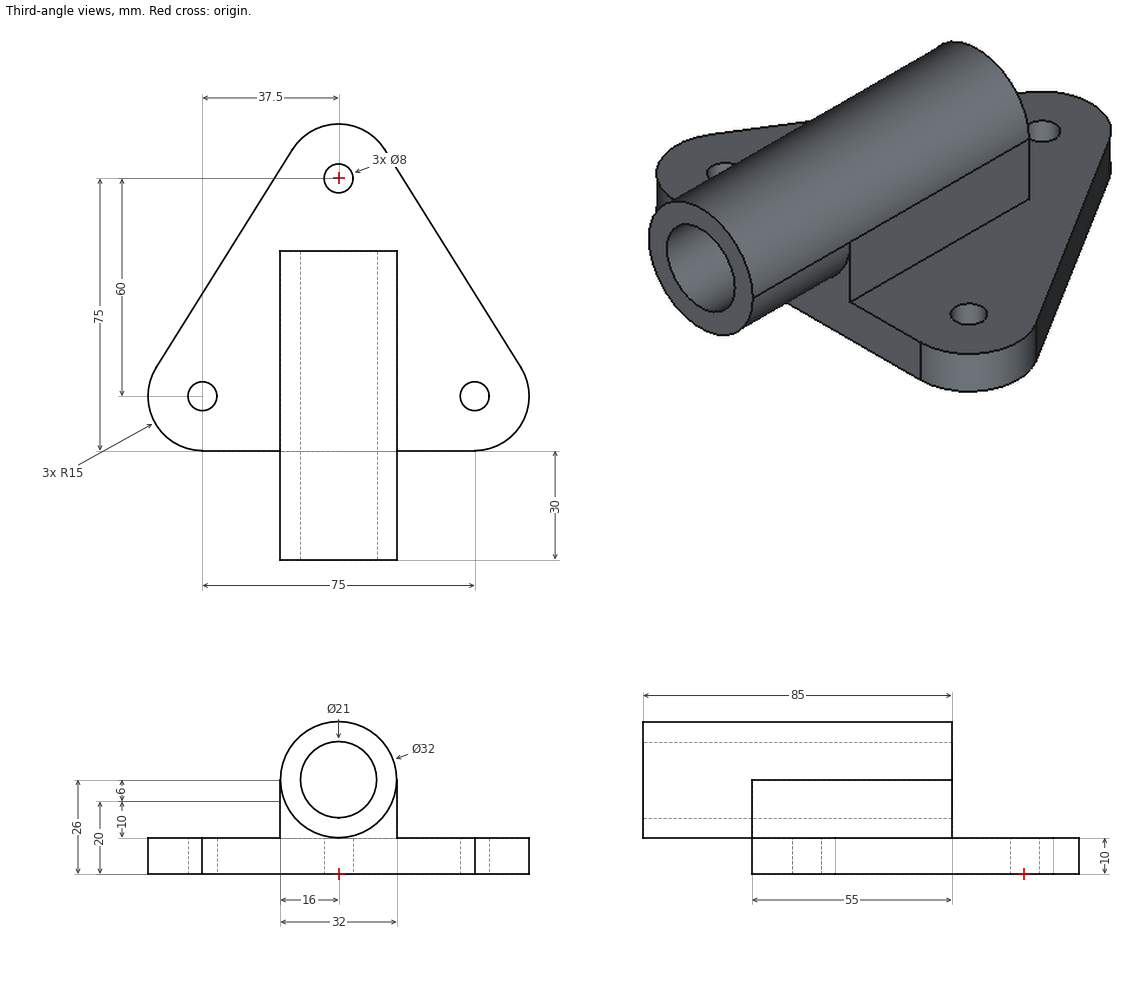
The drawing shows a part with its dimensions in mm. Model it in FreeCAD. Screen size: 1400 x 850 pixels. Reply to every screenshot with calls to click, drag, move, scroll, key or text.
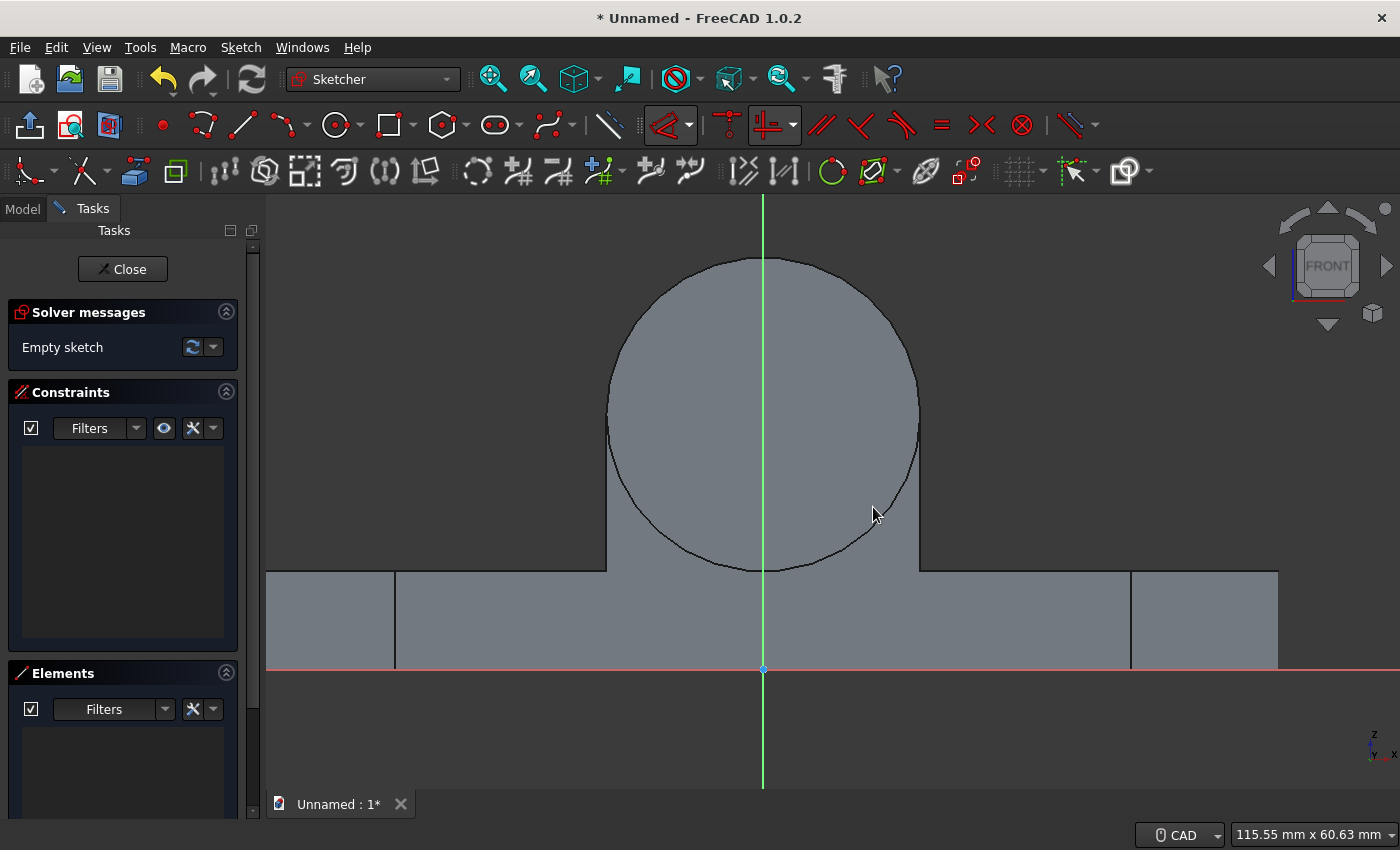
click(336, 126)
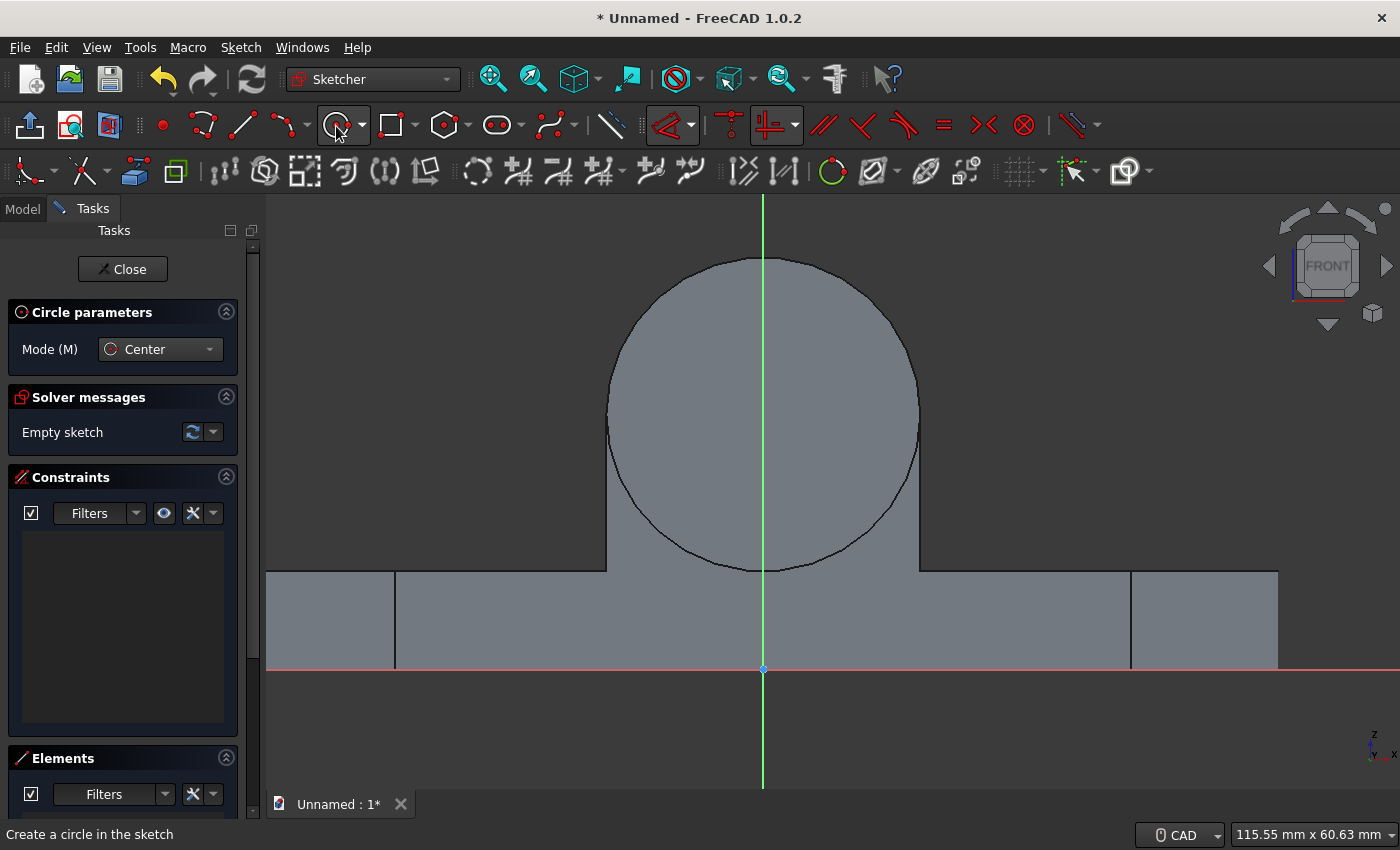
click(763, 414)
click(836, 342)
key(Escape)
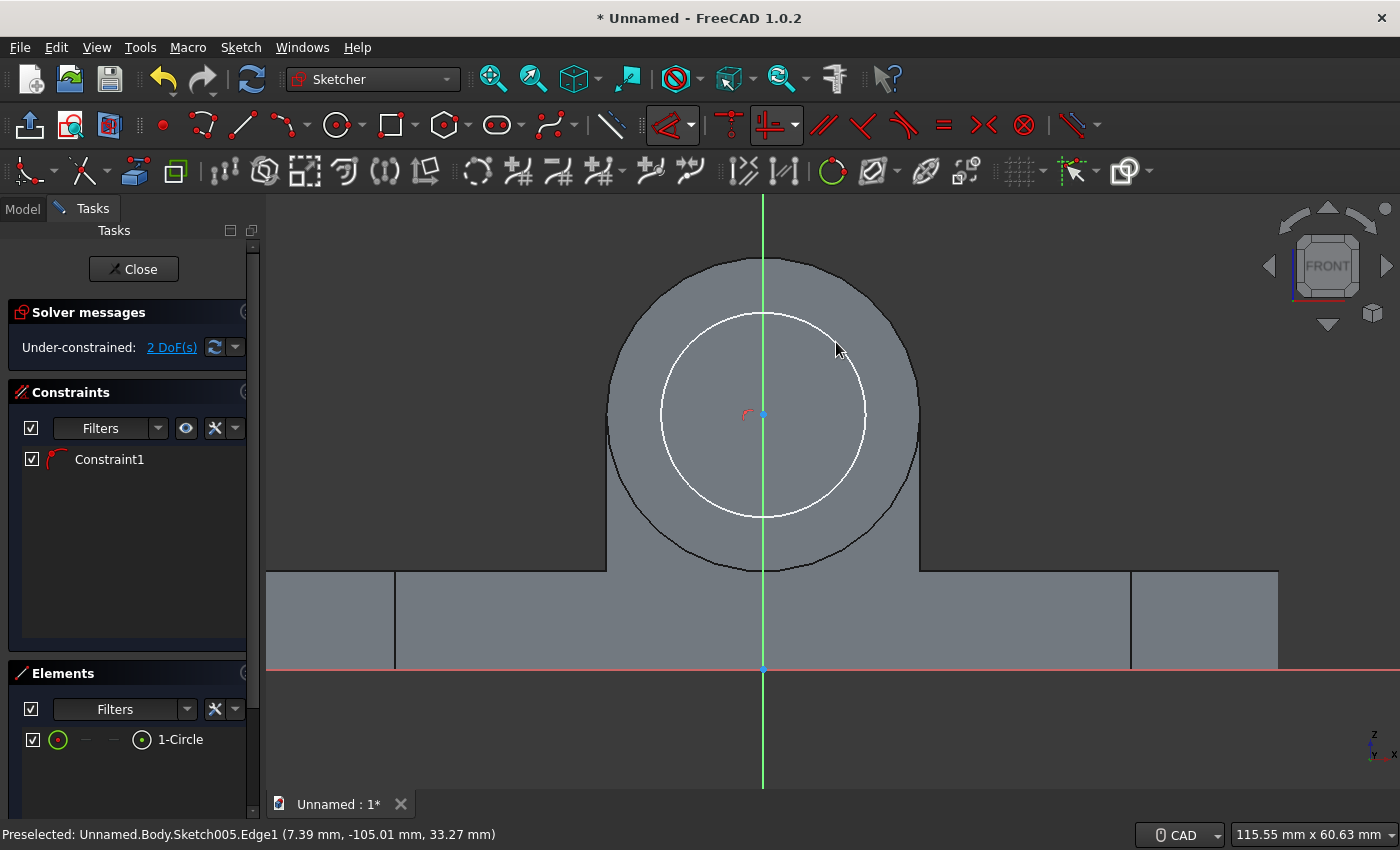
click(835, 342)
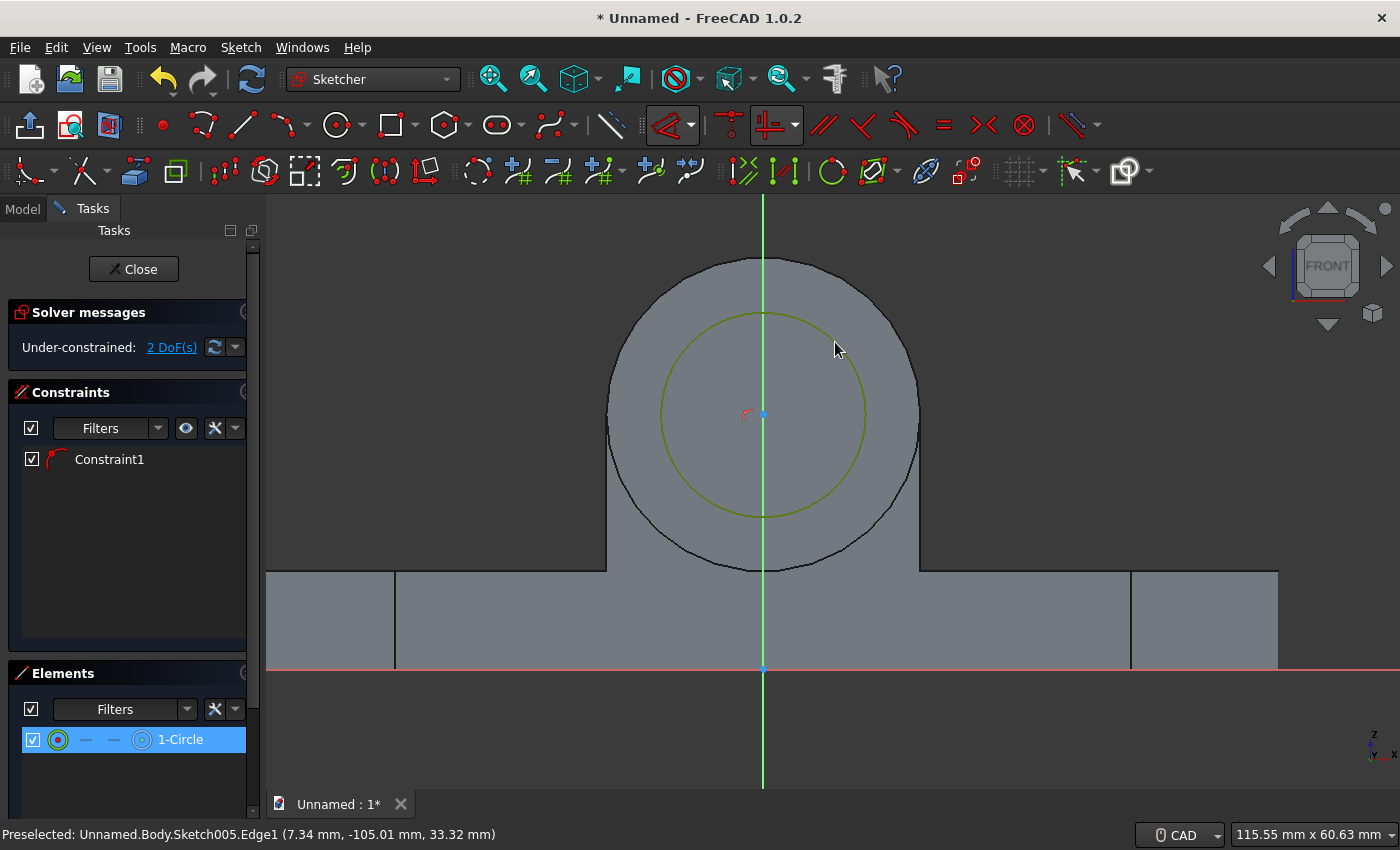
key(k)
key(o)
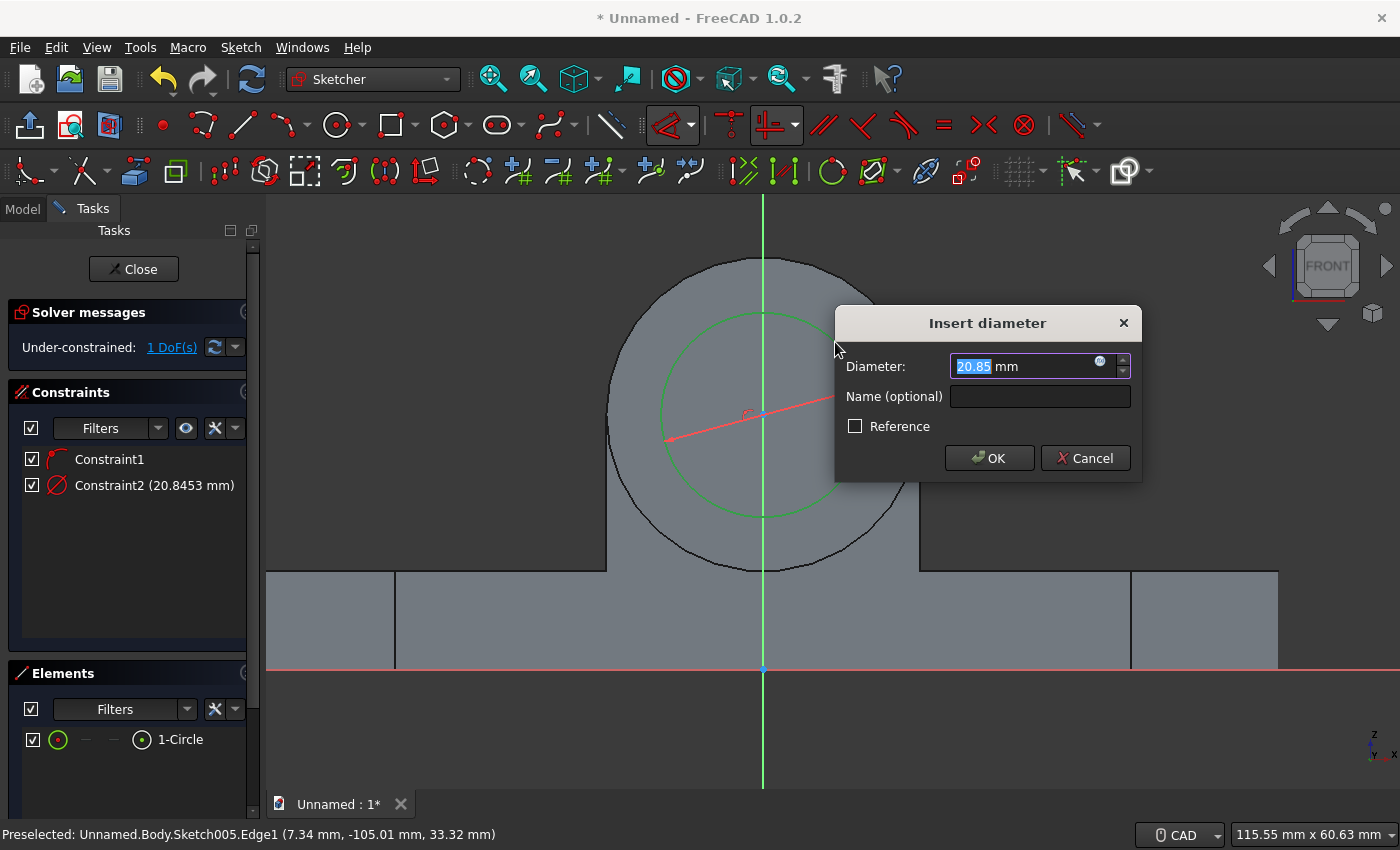
text(21)
key(Return)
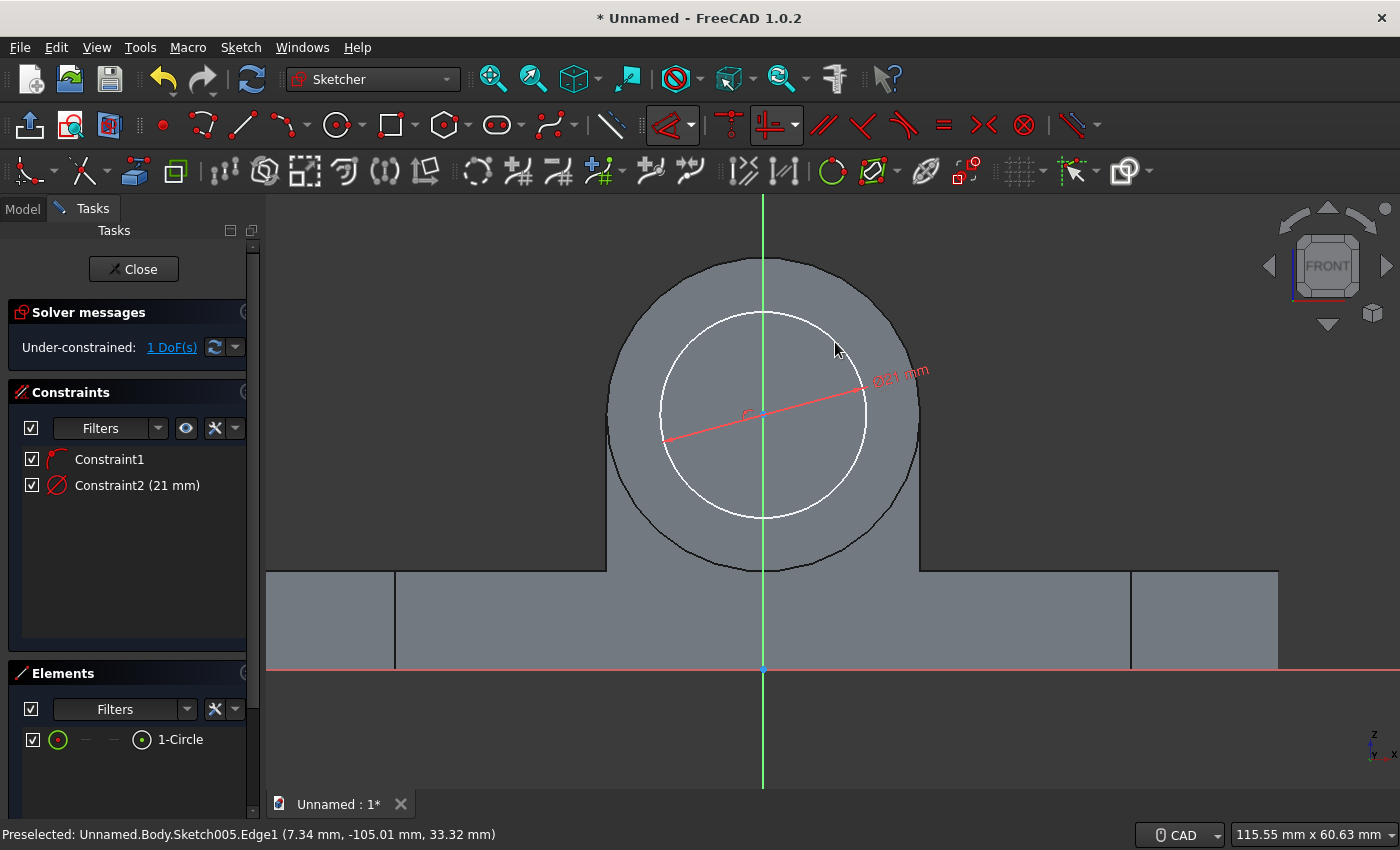
click(763, 415)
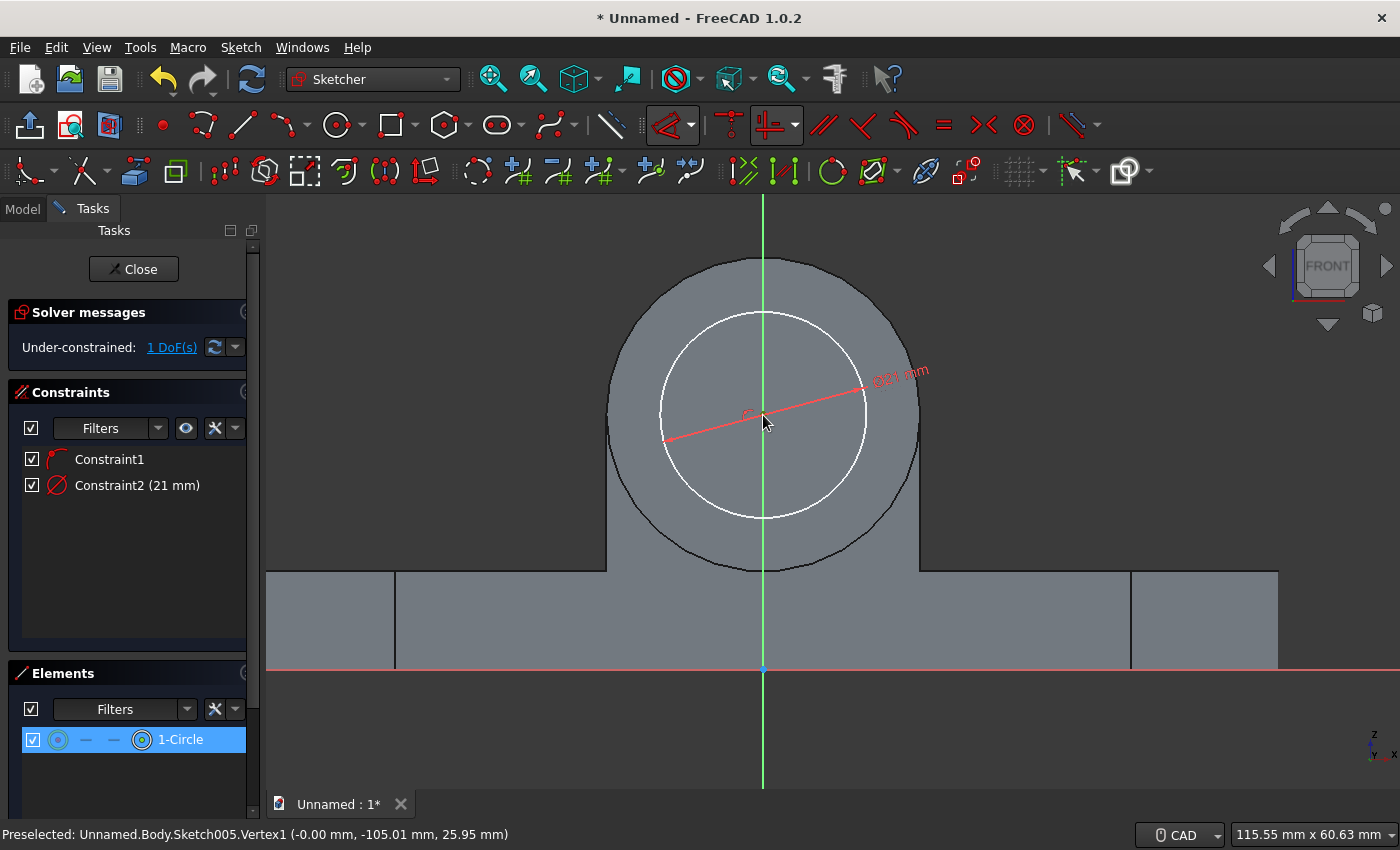
click(694, 126)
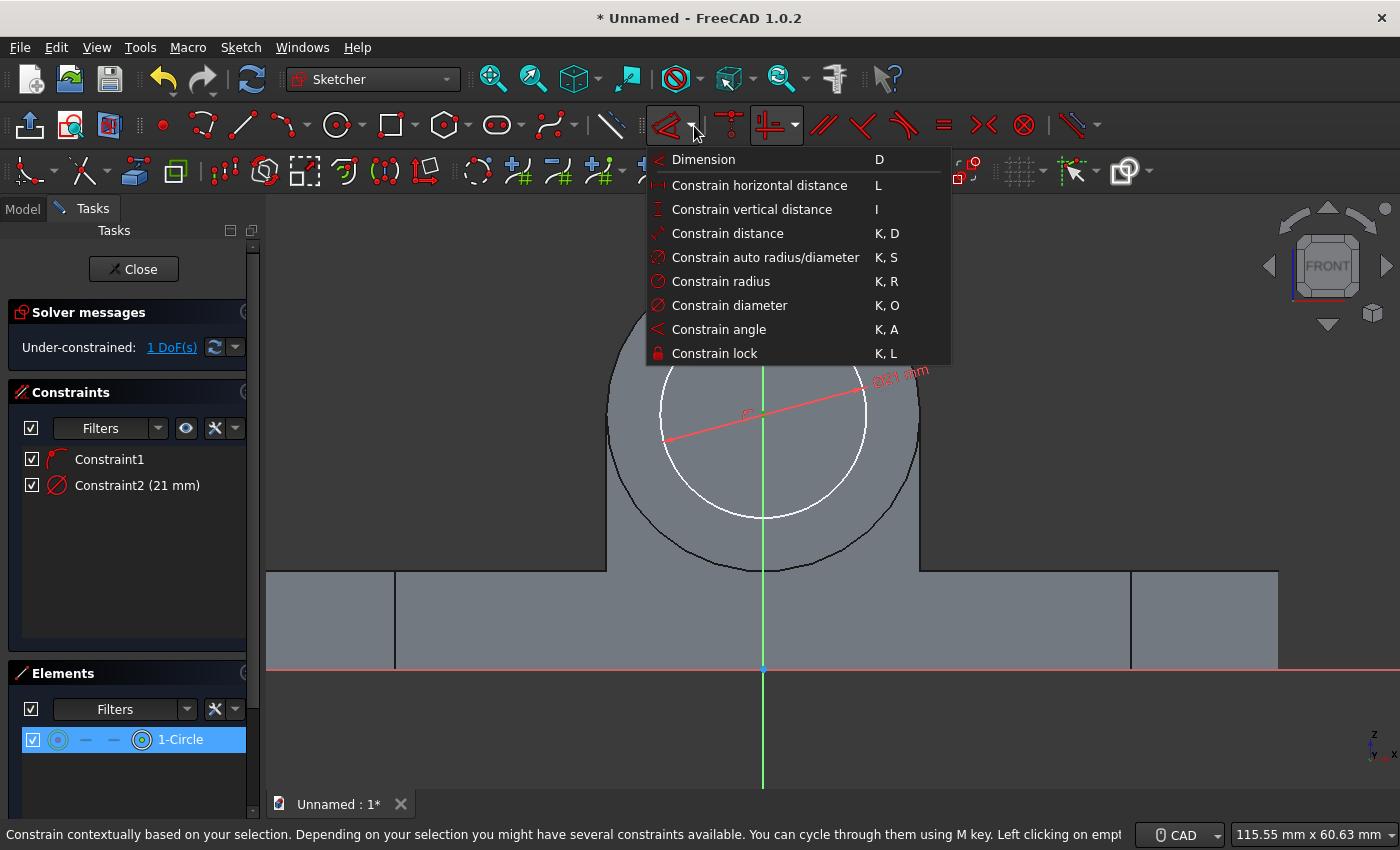
click(799, 209)